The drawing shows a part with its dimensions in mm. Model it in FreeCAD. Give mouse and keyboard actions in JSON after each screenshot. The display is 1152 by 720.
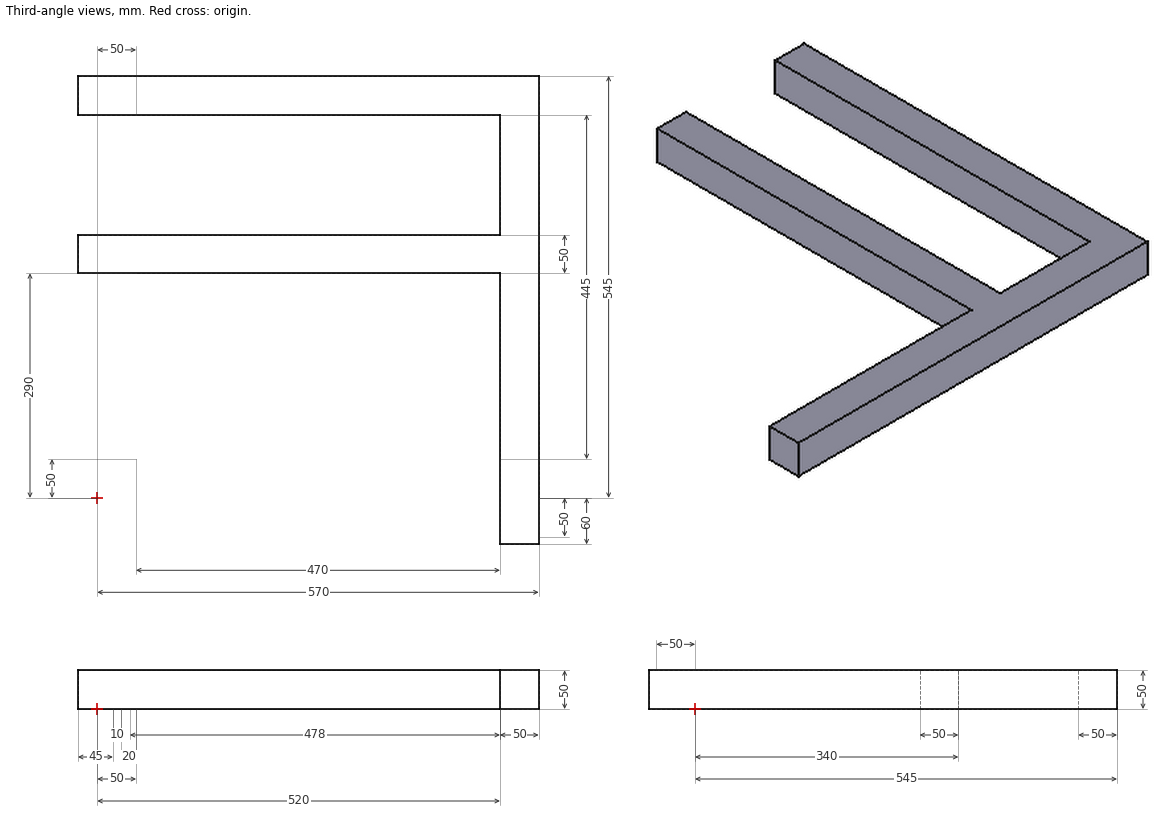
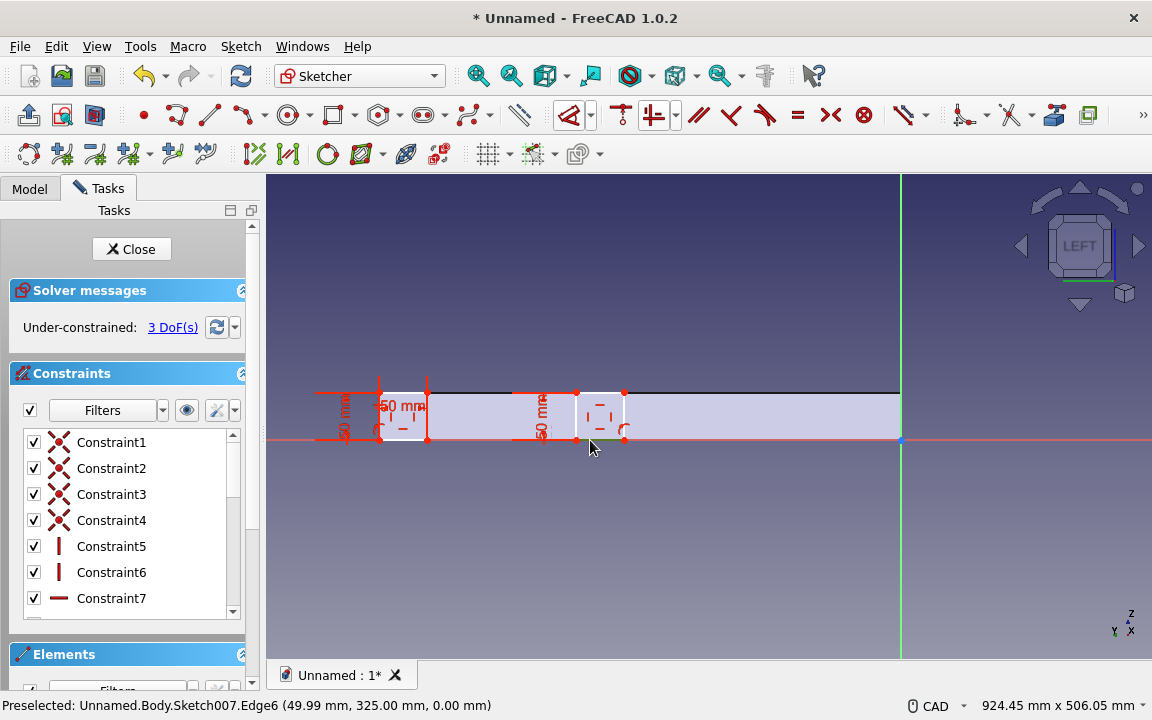
{"action": "key", "text": "l"}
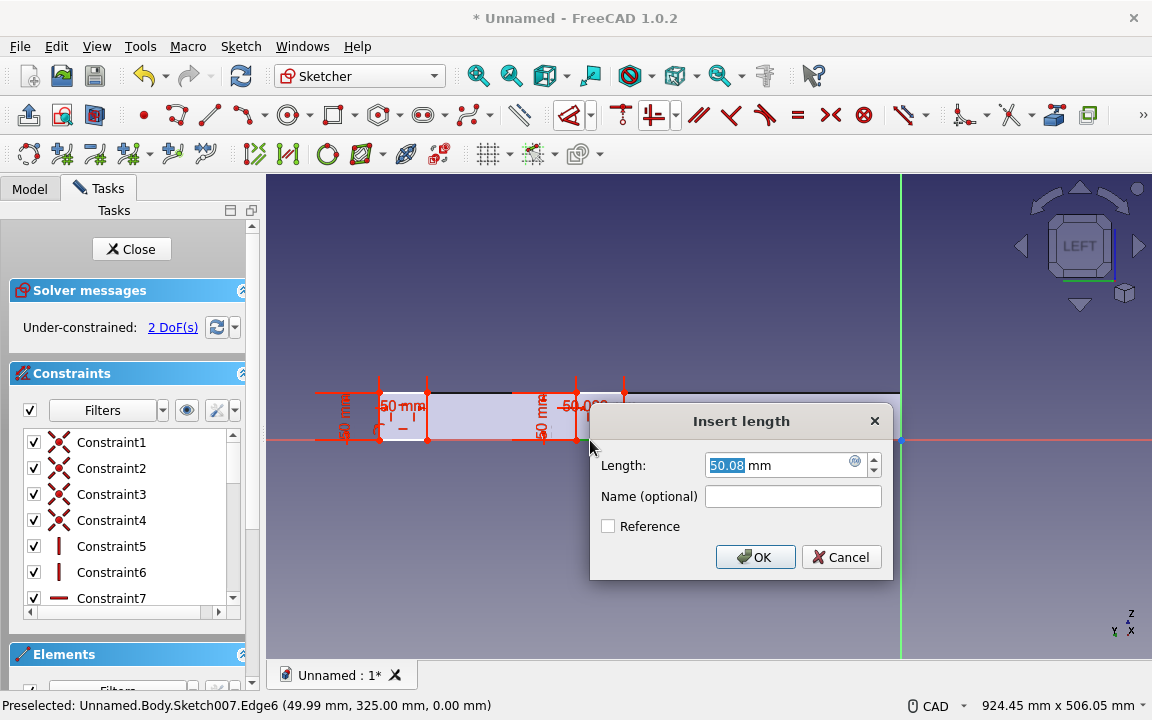
{"action": "type", "text": "50"}
{"action": "key", "text": "Return"}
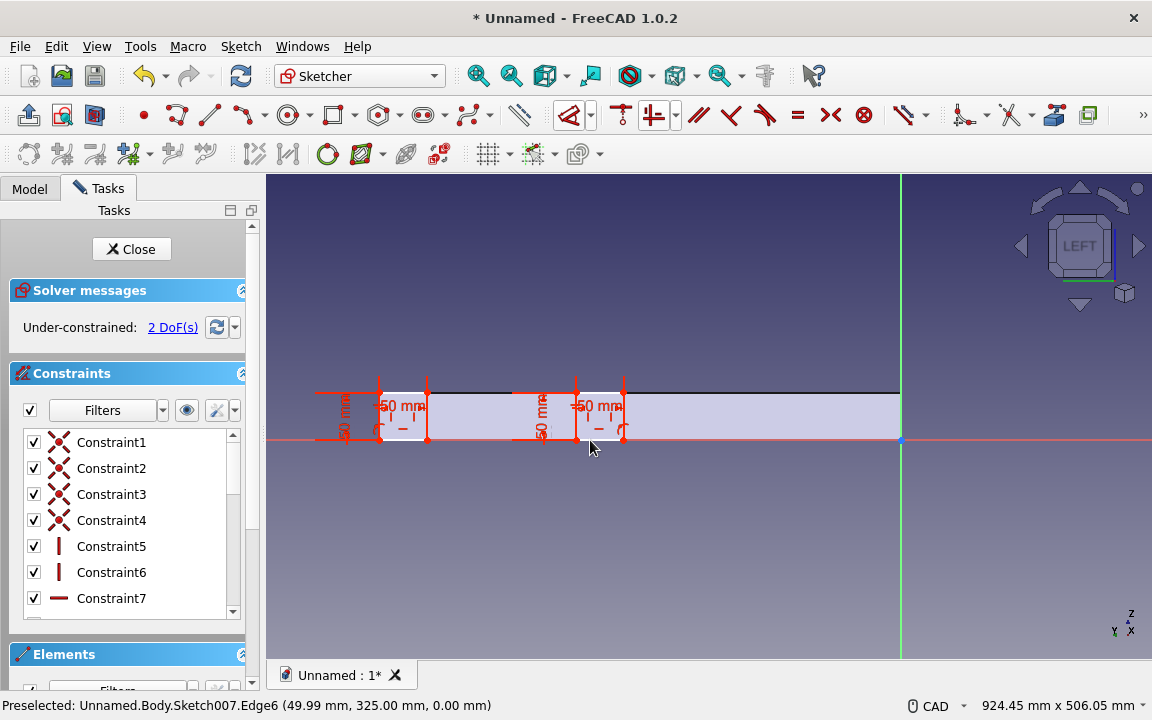
{"action": "left_click", "coordinate": [379, 393]}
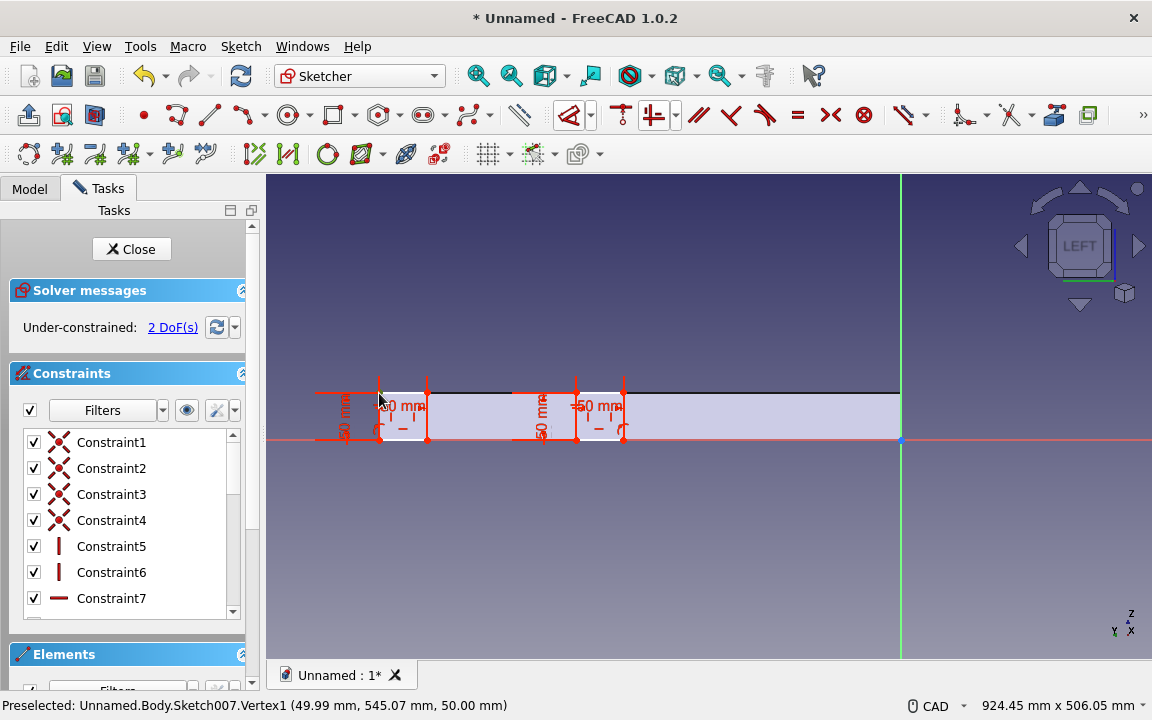
{"action": "left_click", "coordinate": [590, 116]}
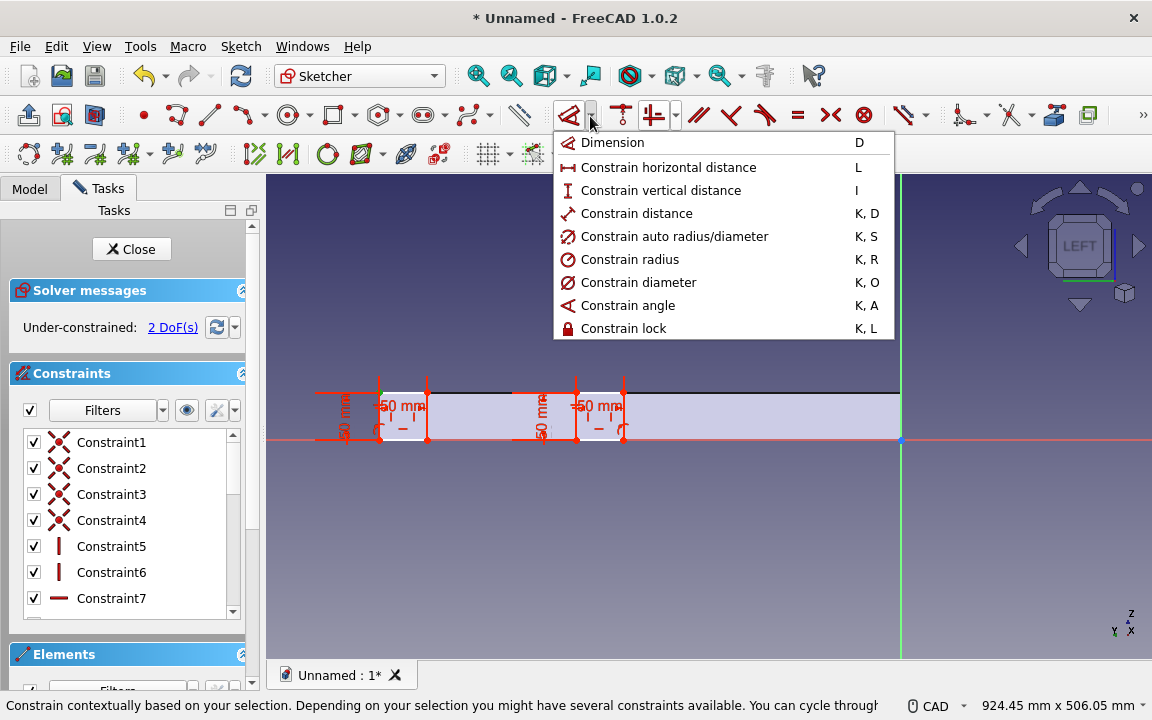
{"action": "left_click", "coordinate": [724, 168]}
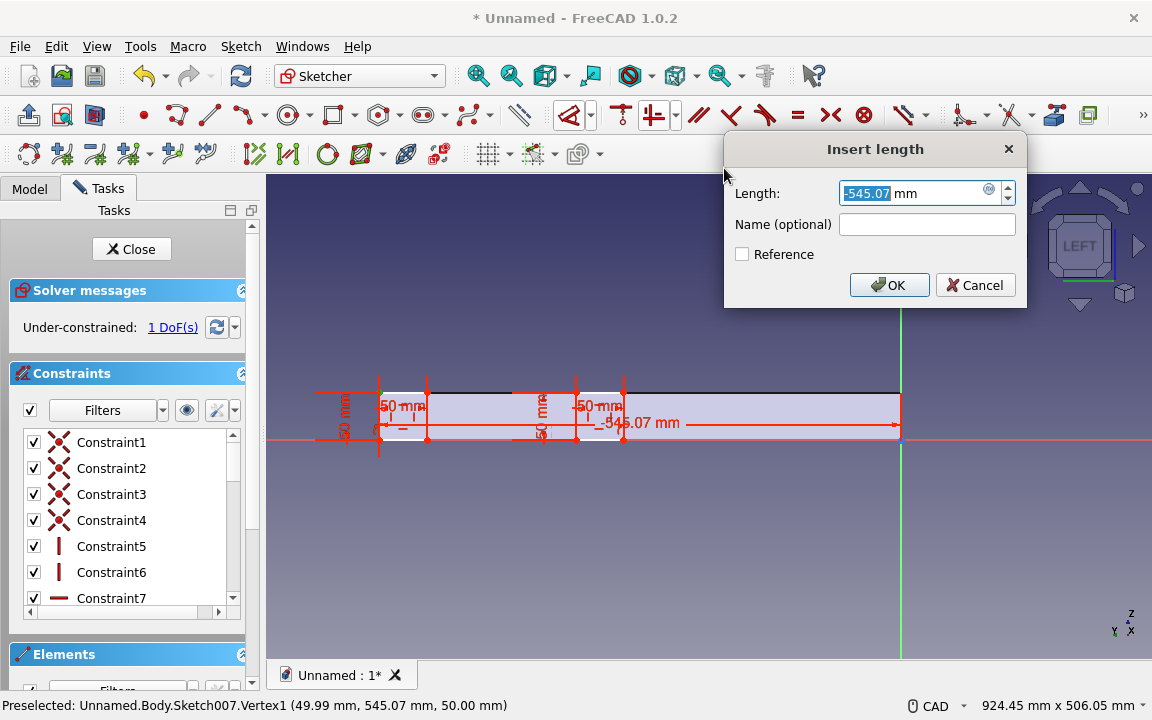
{"action": "type", "text": "-545"}
{"action": "key", "text": "Return"}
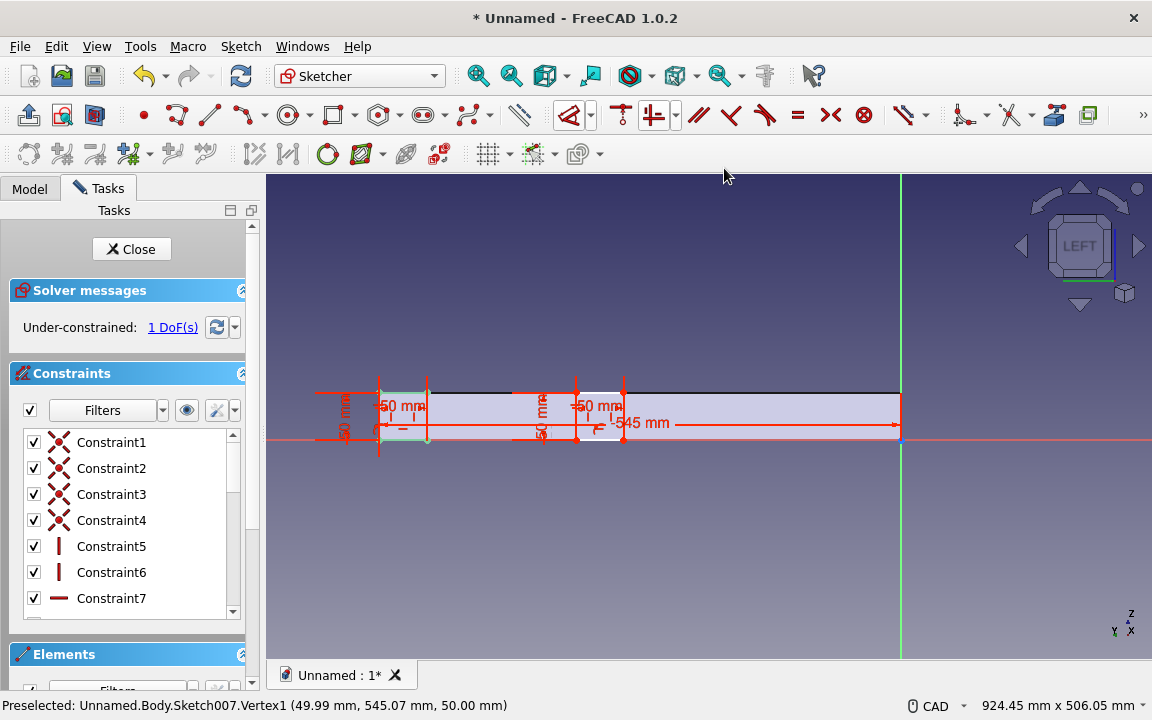
{"action": "left_click", "coordinate": [576, 393]}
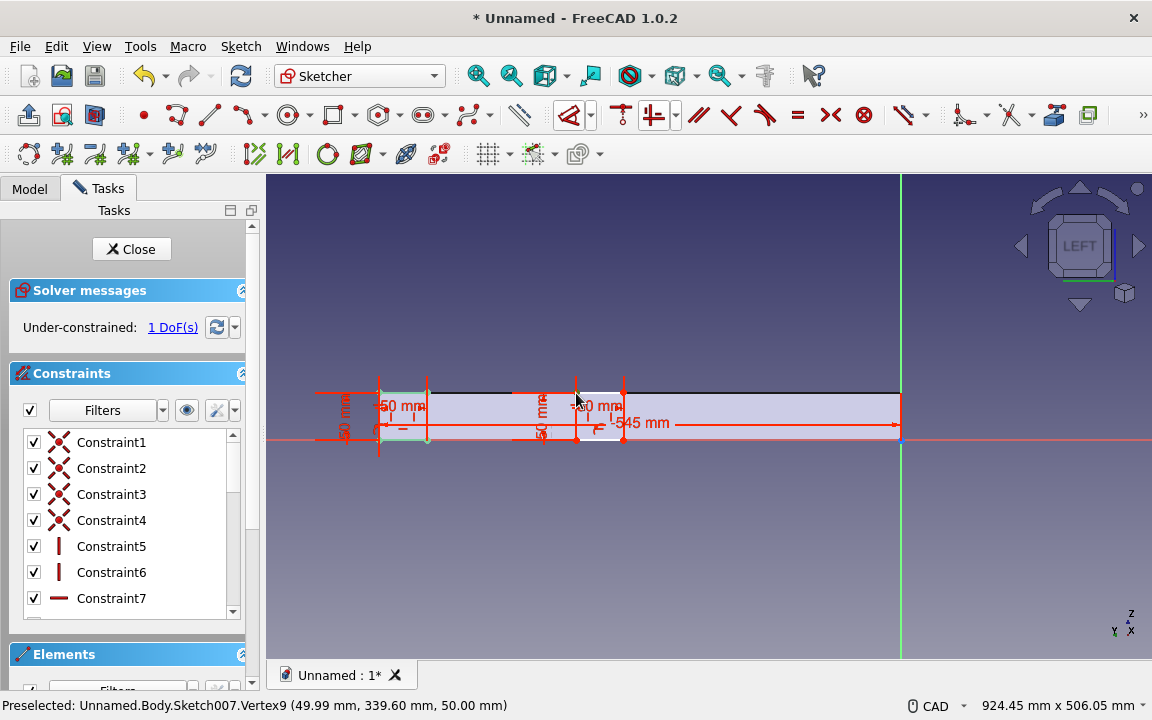
{"action": "key", "text": "l"}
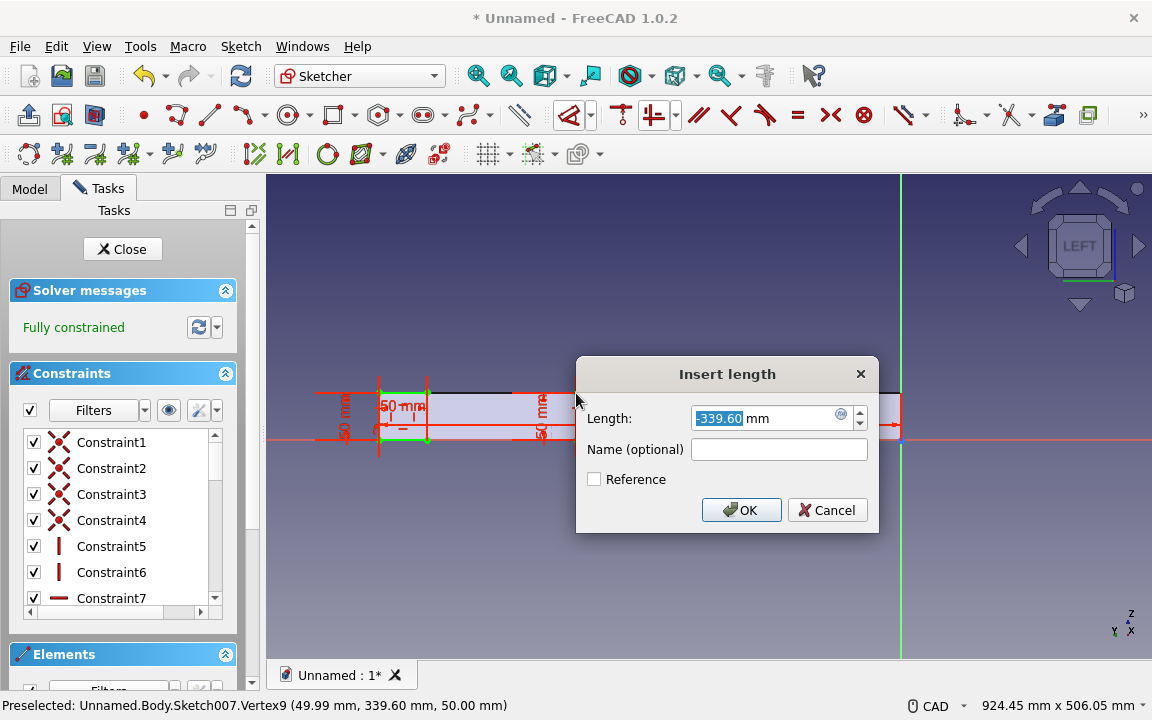
{"action": "type", "text": "-340"}
{"action": "key", "text": "Return"}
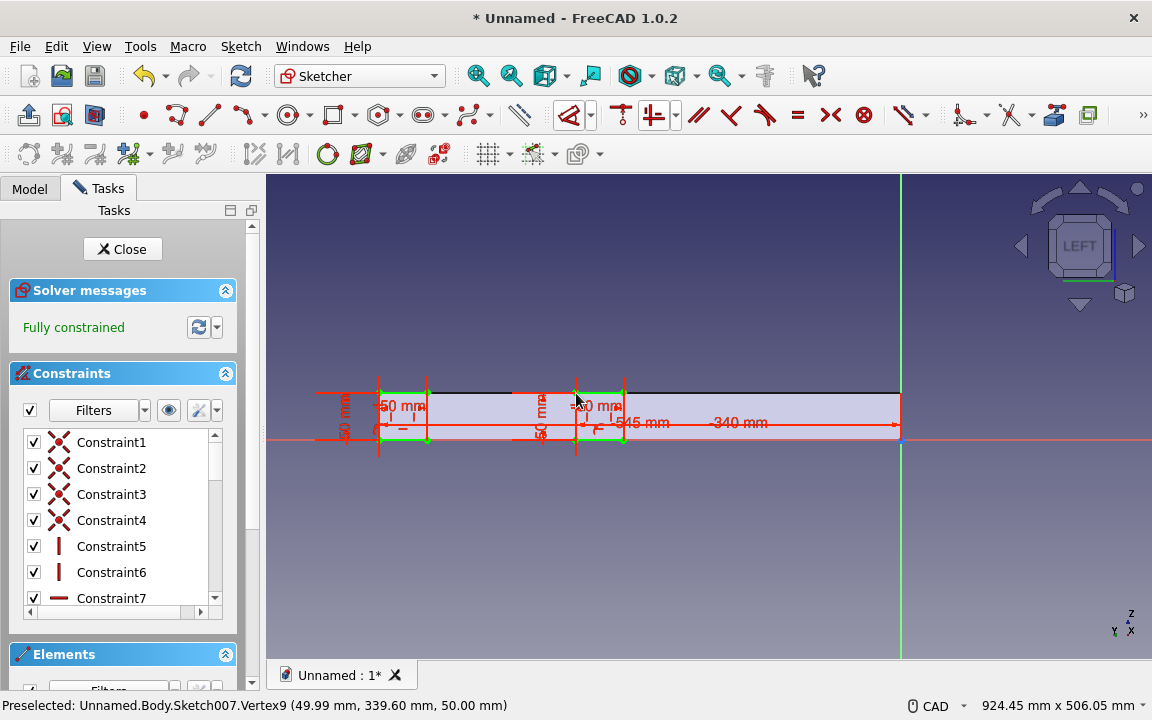
{"action": "left_click", "coordinate": [123, 249]}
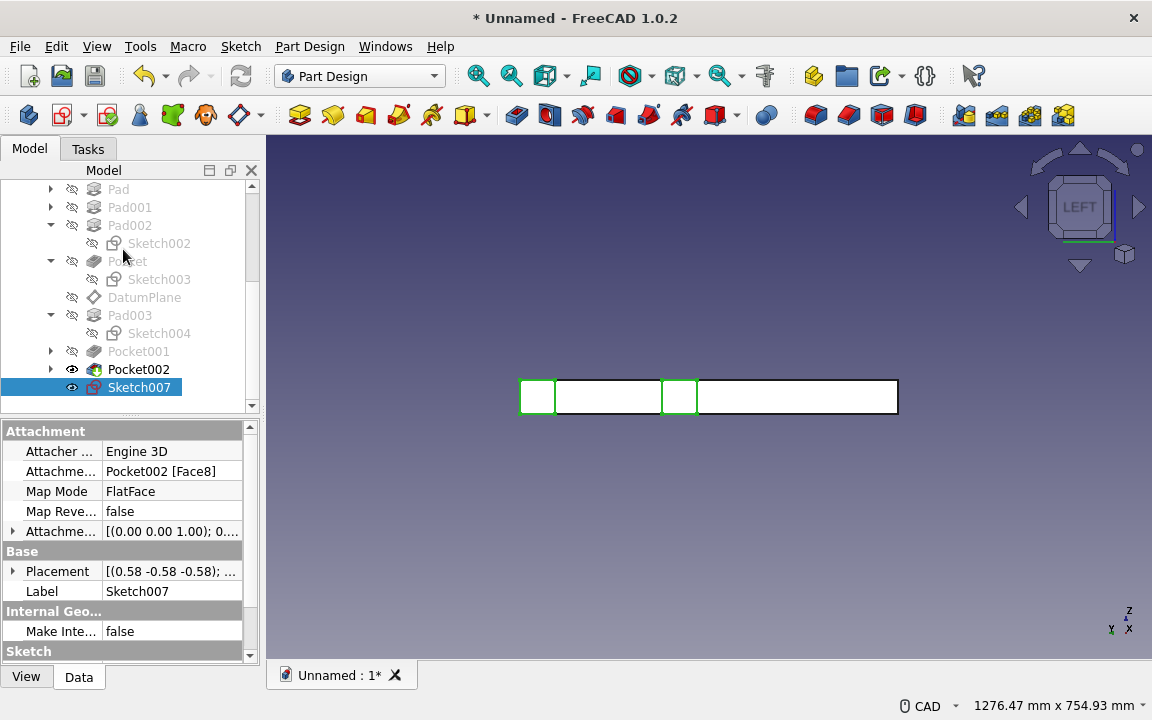
{"action": "left_click", "coordinate": [300, 116]}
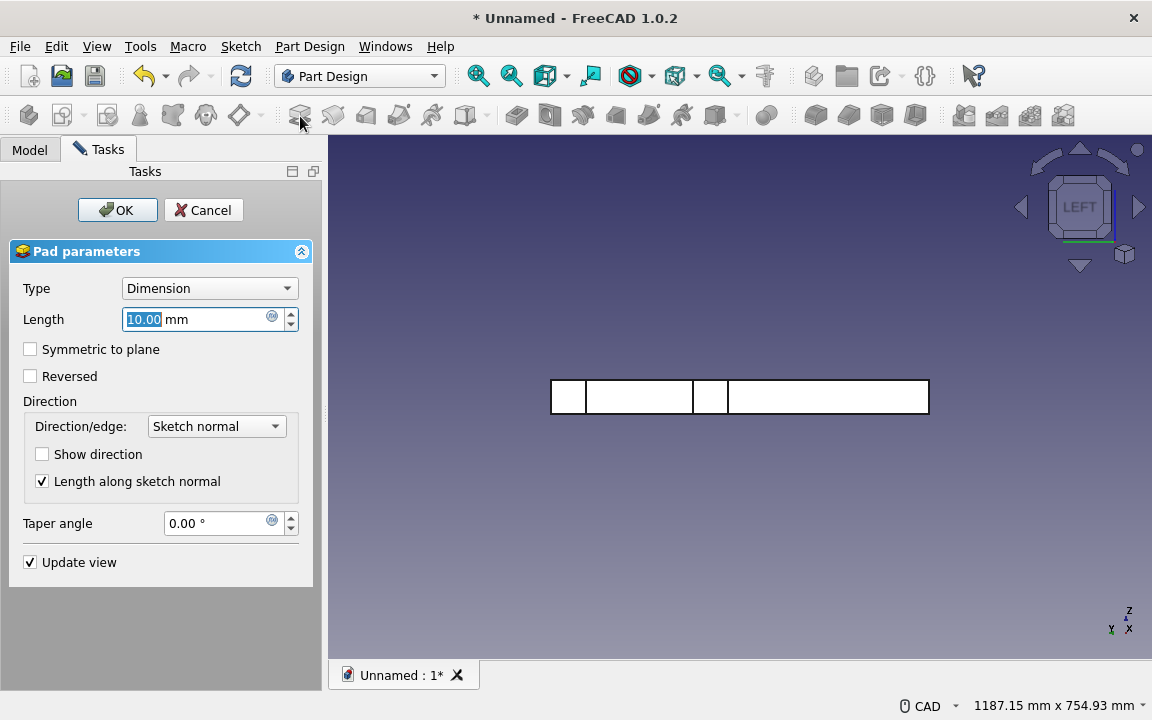
{"action": "type", "text": "20"}
{"action": "key", "text": "Tab"}